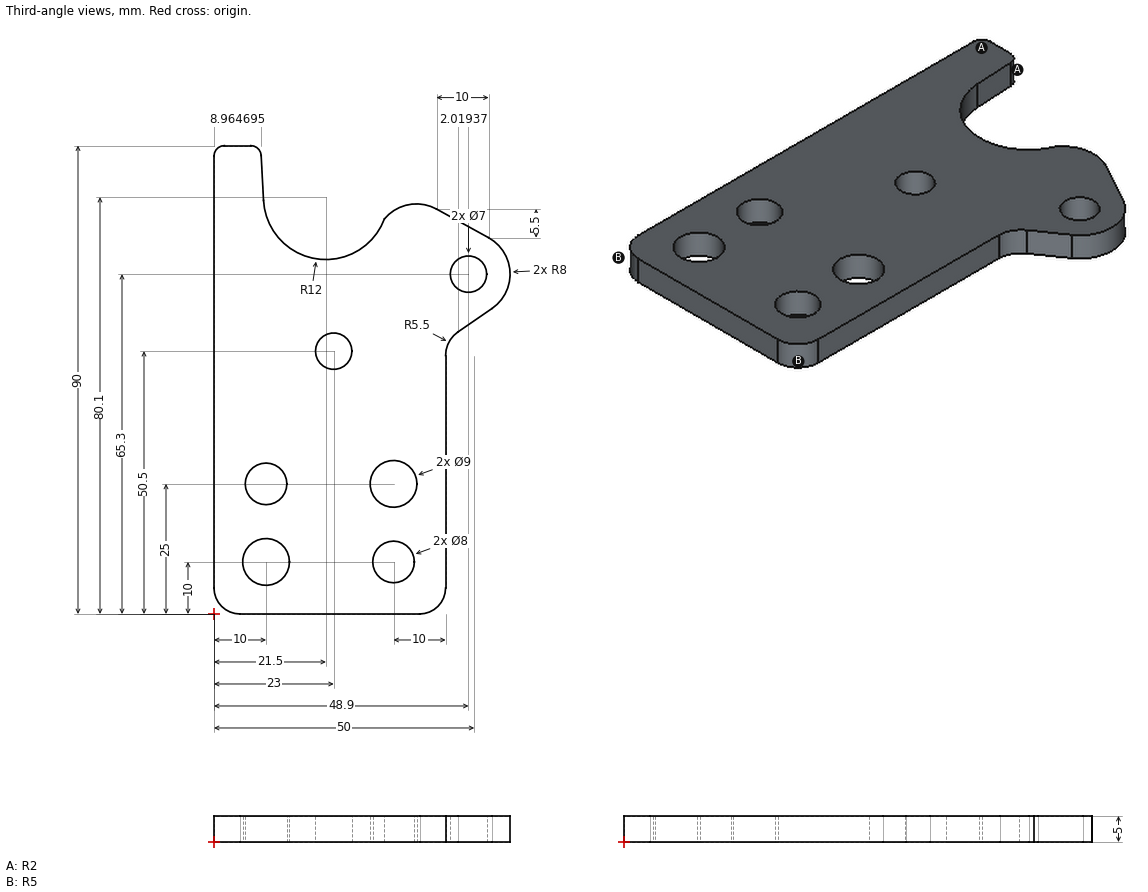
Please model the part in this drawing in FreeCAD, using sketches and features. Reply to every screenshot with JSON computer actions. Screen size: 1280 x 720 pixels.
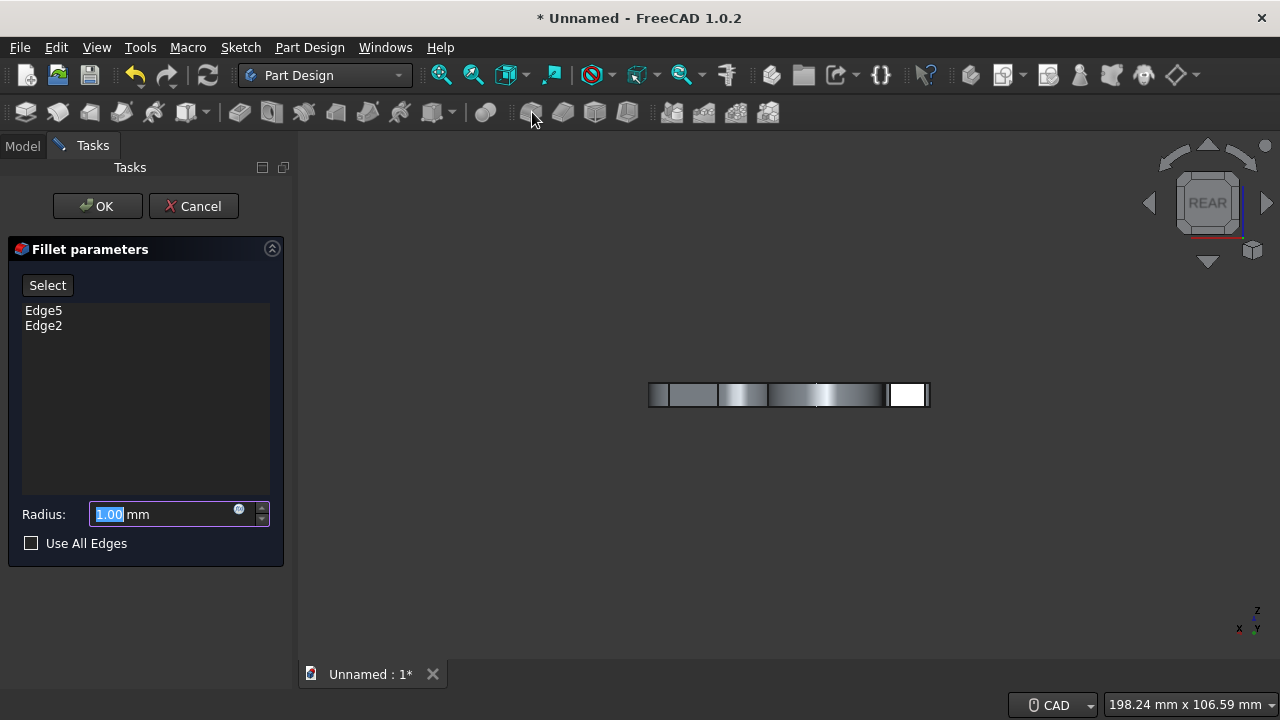
{"action": "type", "text": "2"}
{"action": "key", "text": "Tab"}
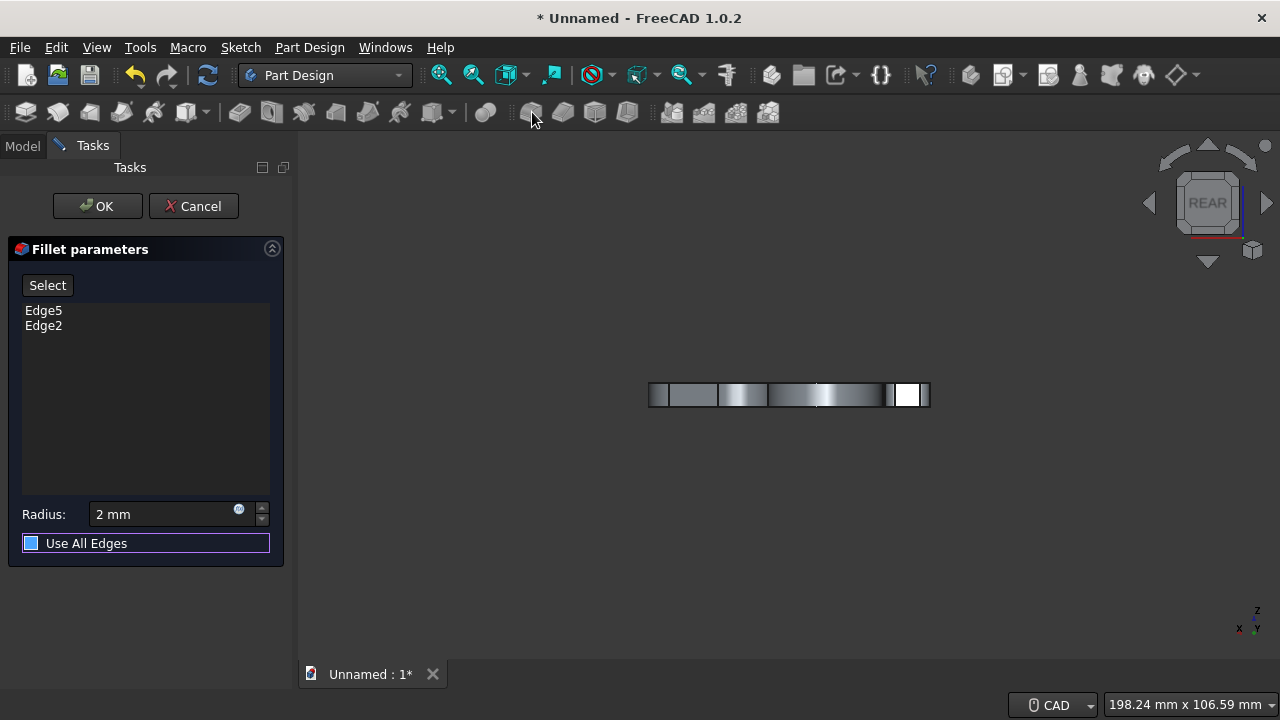
{"action": "left_click", "coordinate": [98, 206]}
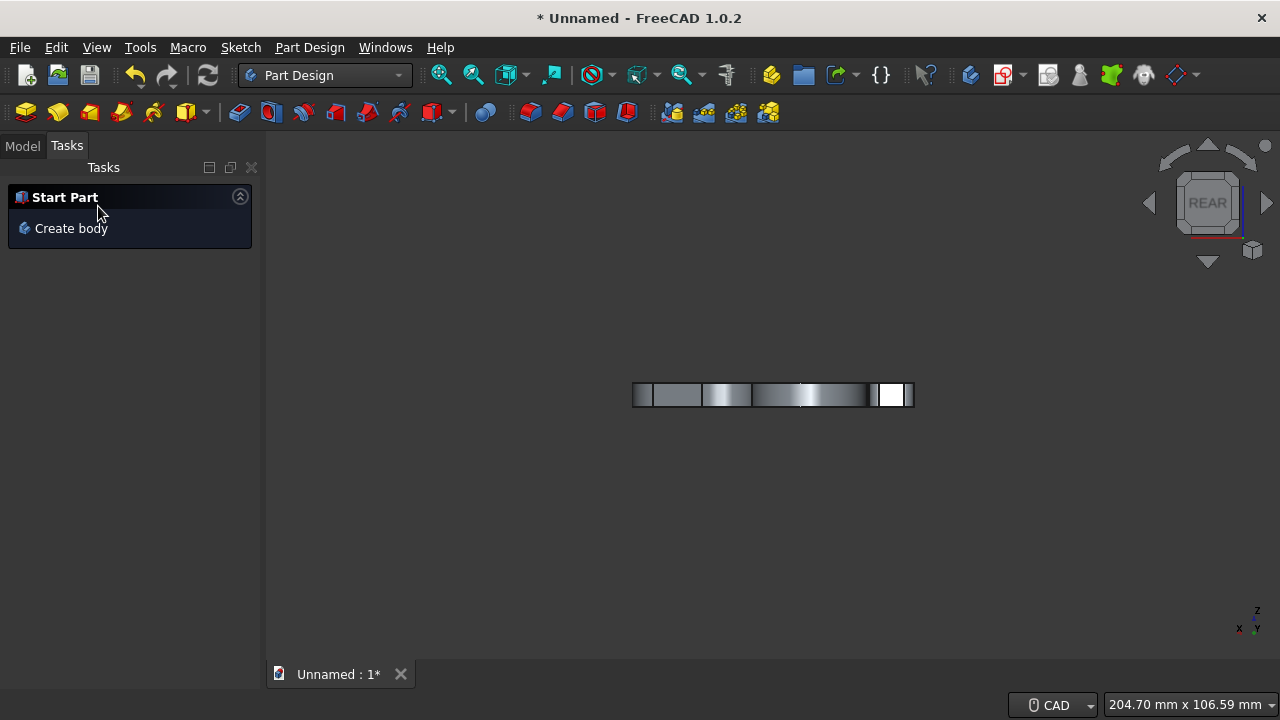
{"action": "key", "text": "v f"}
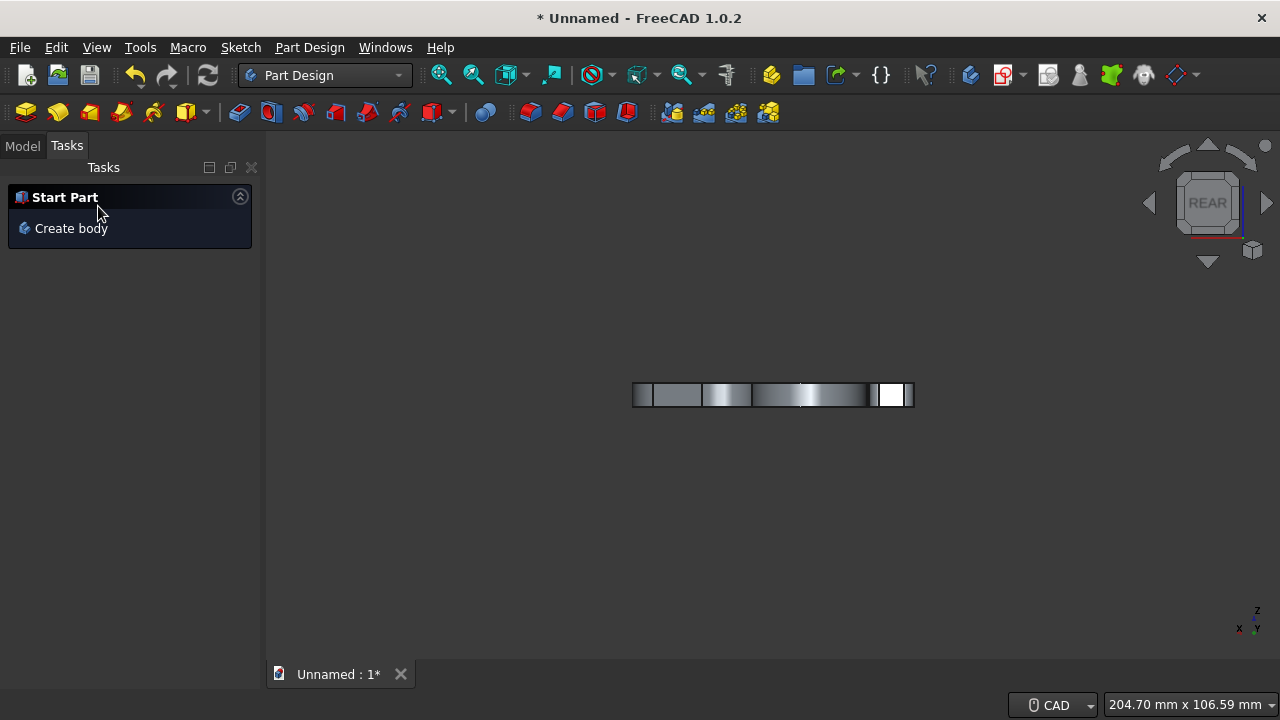
{"action": "key", "text": "0"}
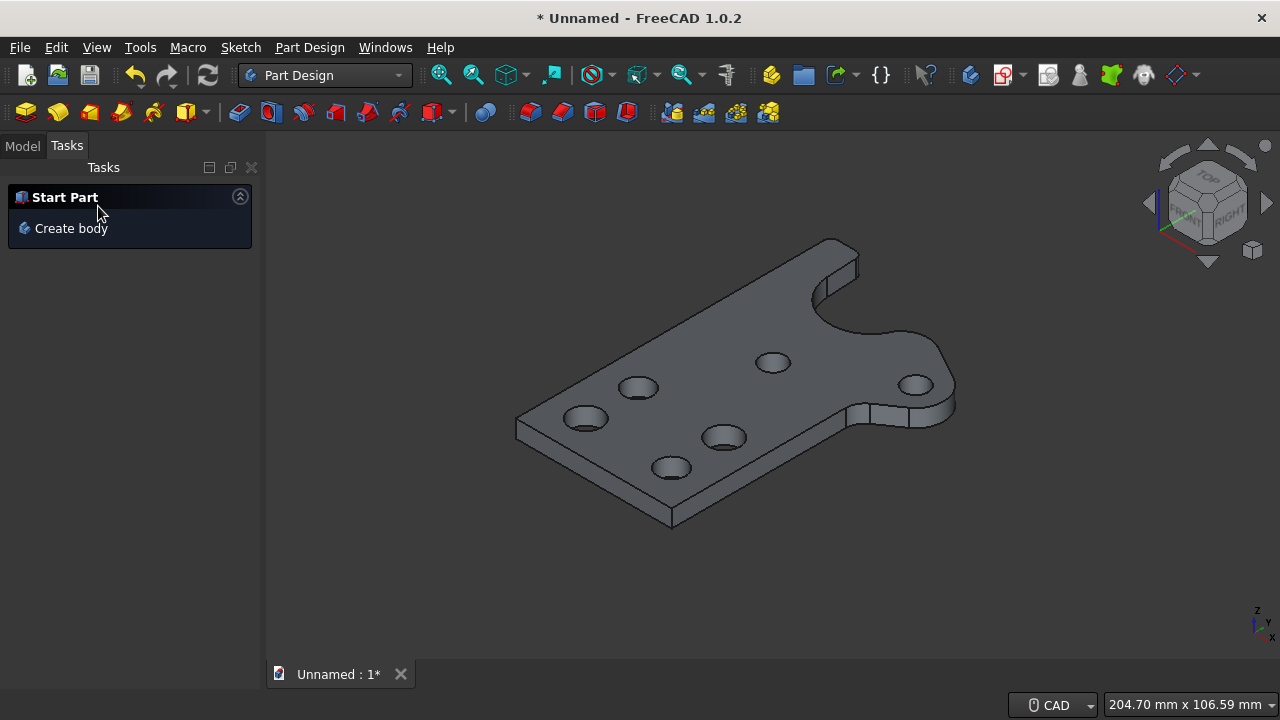
{"action": "left_click", "coordinate": [672, 517]}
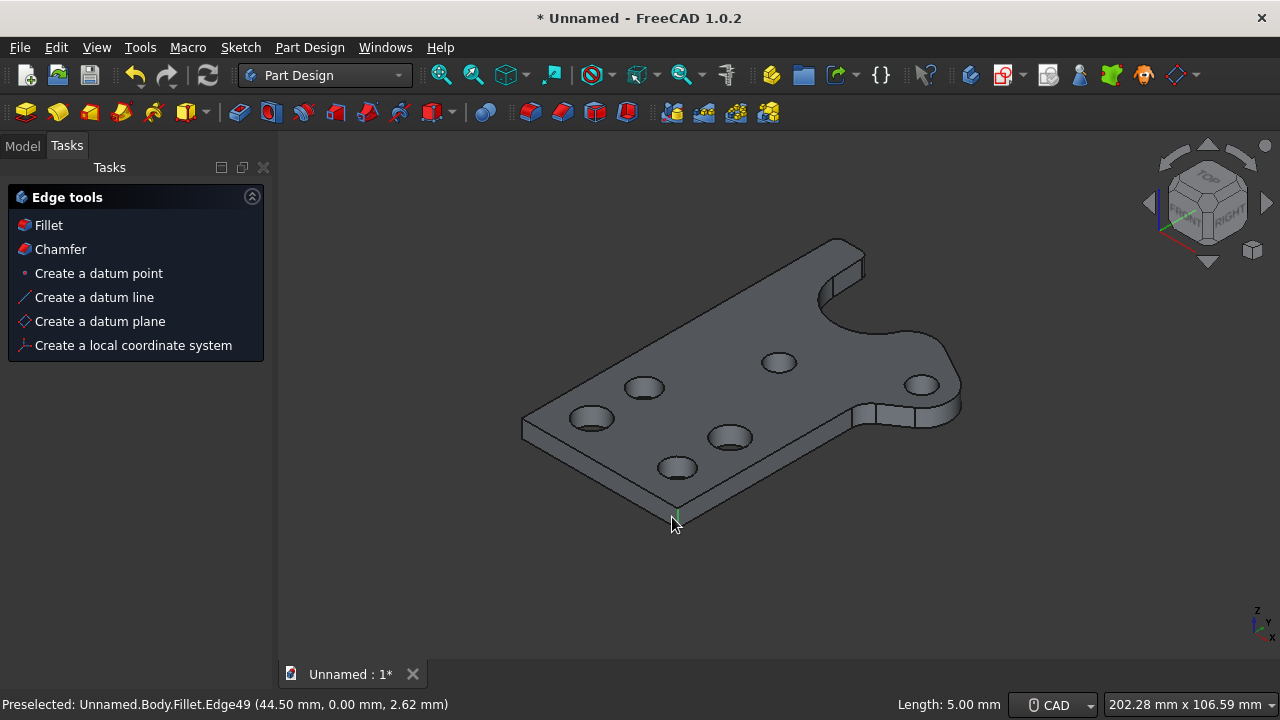
{"action": "key", "text": "2"}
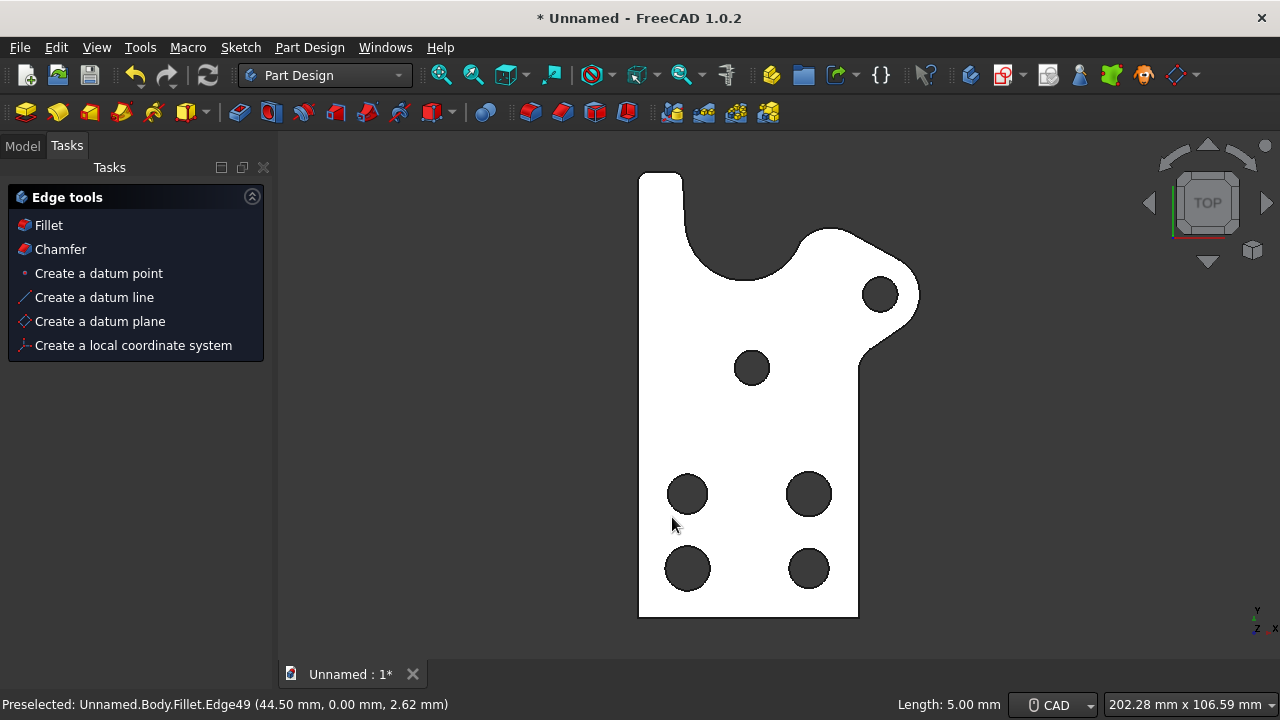
{"action": "key", "text": "1"}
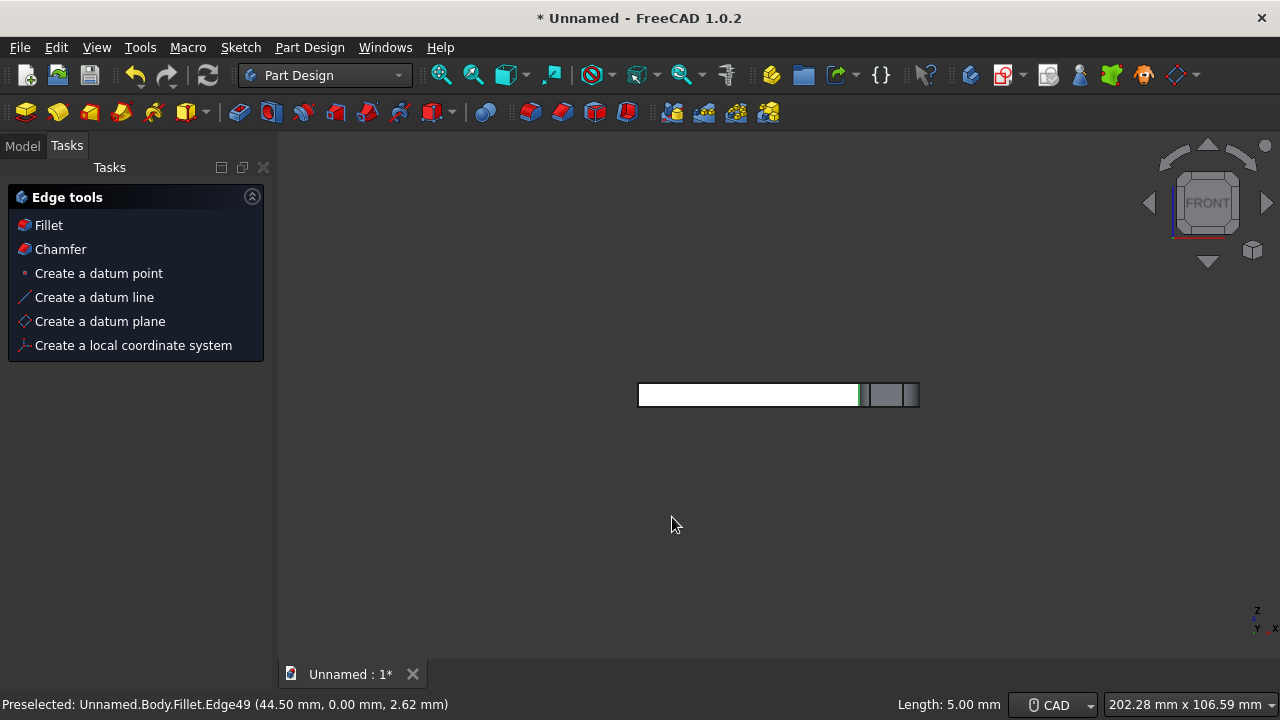
{"action": "key", "text": "v f"}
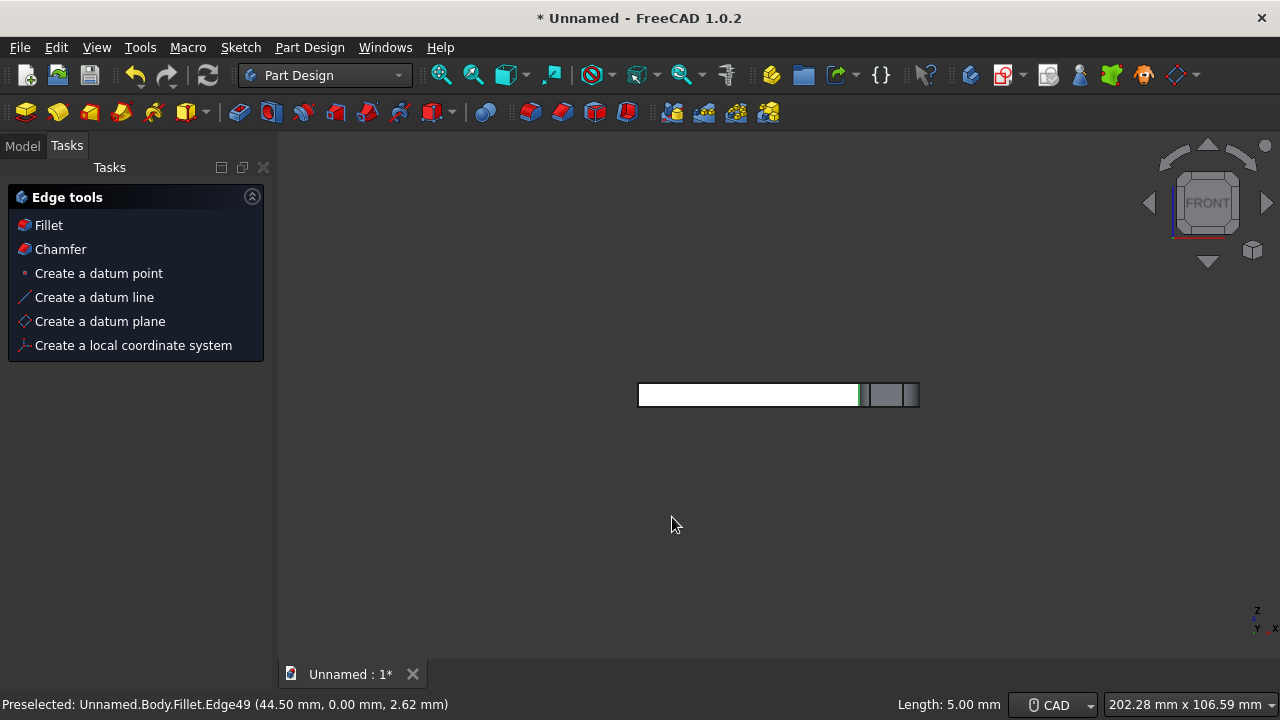
{"action": "left_click", "coordinate": [638, 394], "text": "ctrl"}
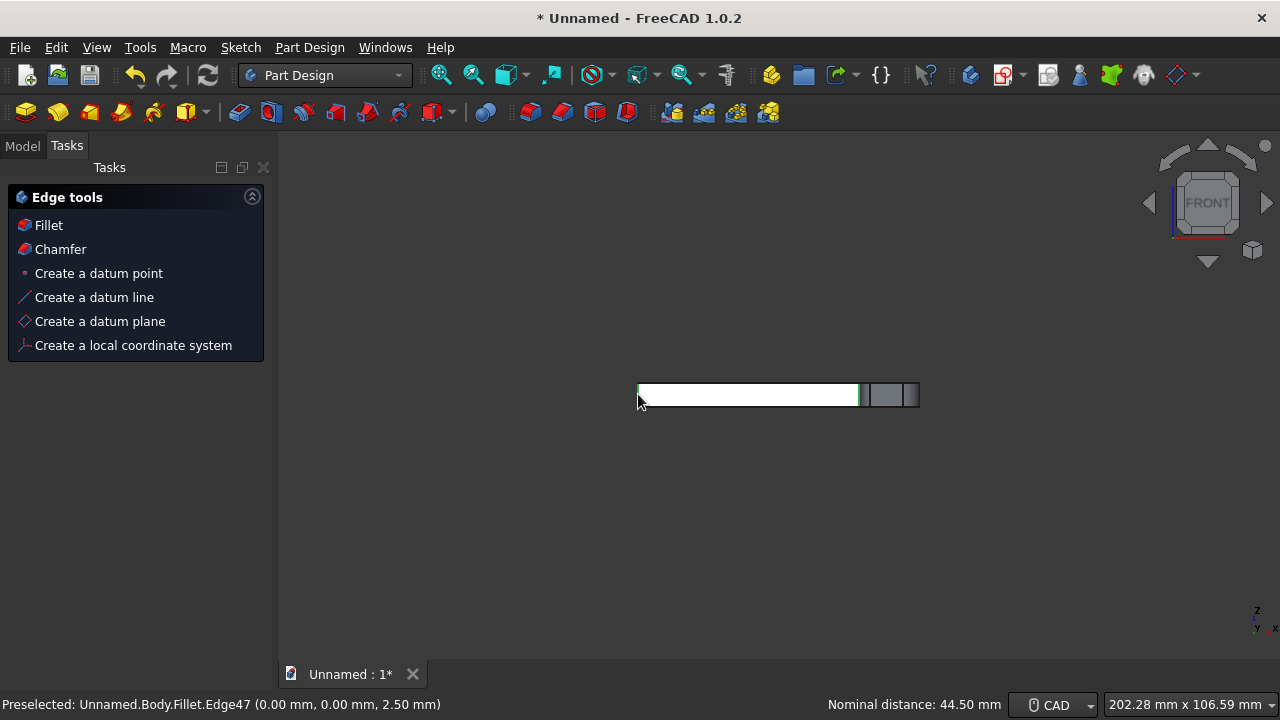
{"action": "left_click", "coordinate": [532, 112]}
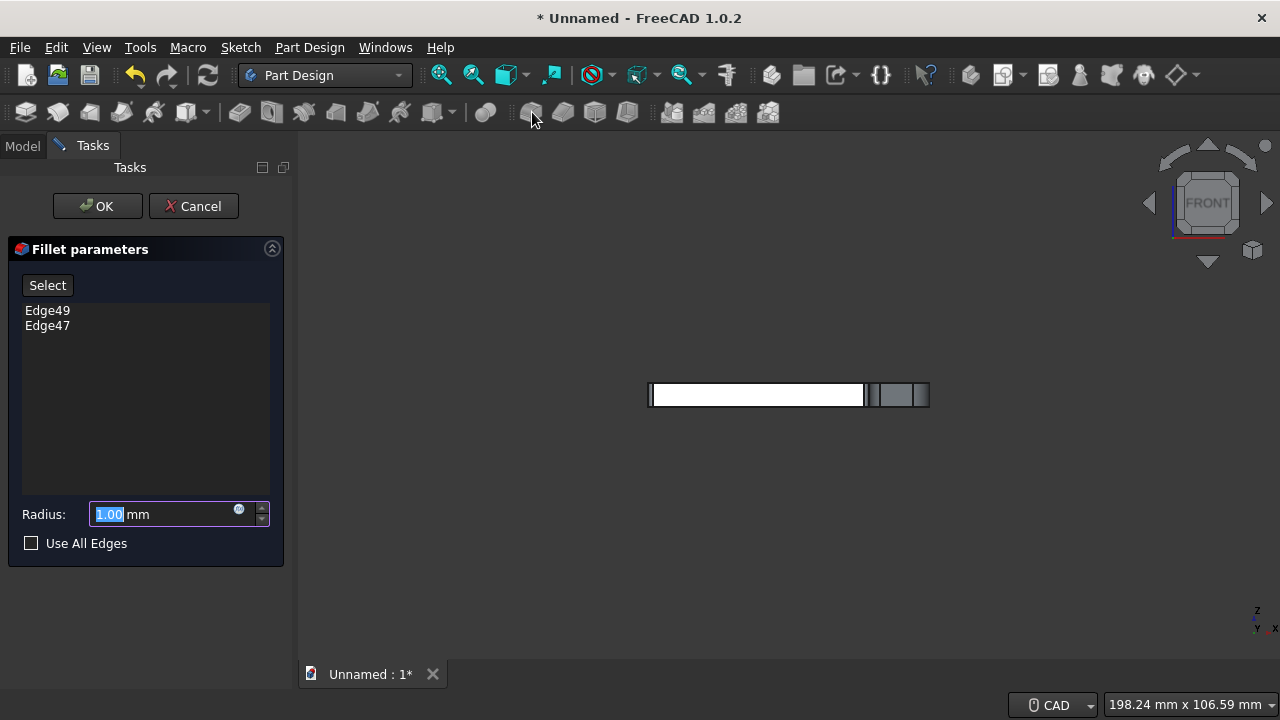
{"action": "type", "text": "5"}
{"action": "key", "text": "Tab"}